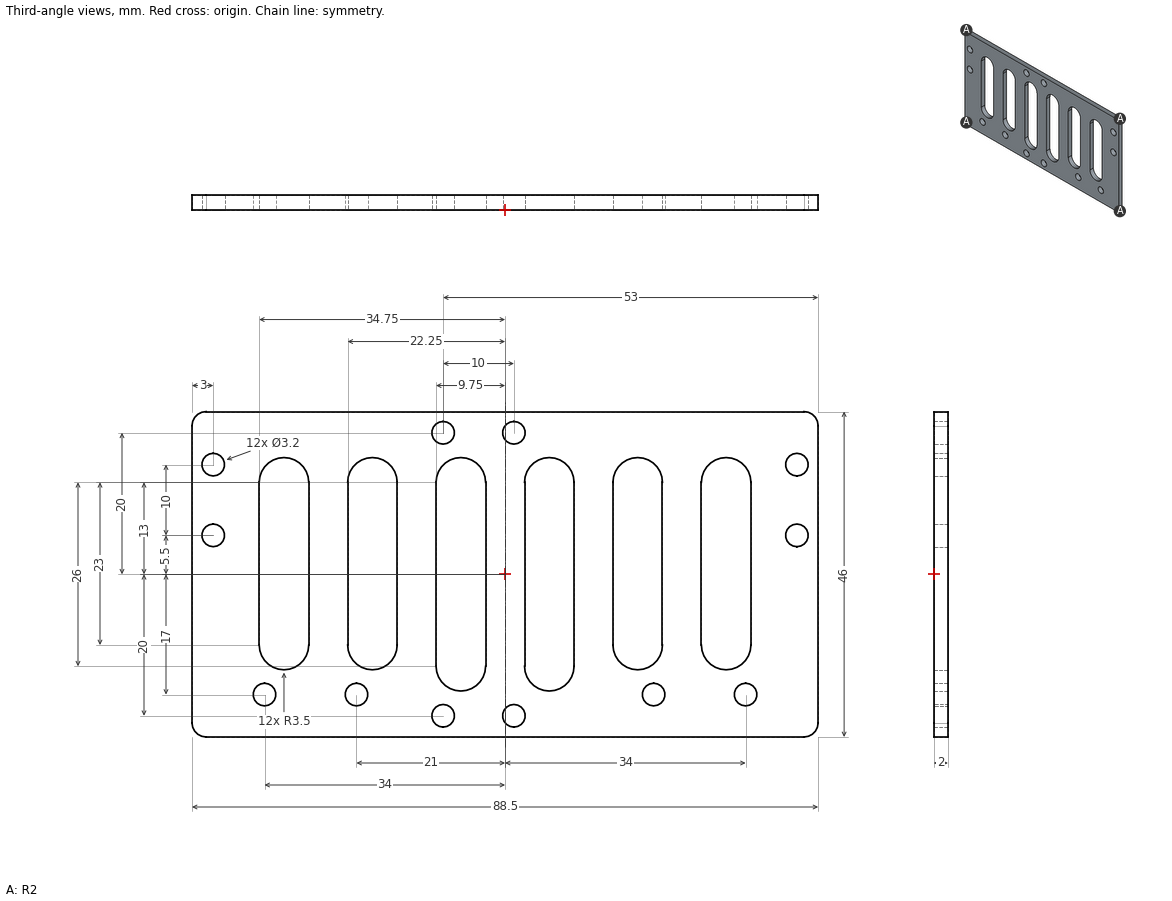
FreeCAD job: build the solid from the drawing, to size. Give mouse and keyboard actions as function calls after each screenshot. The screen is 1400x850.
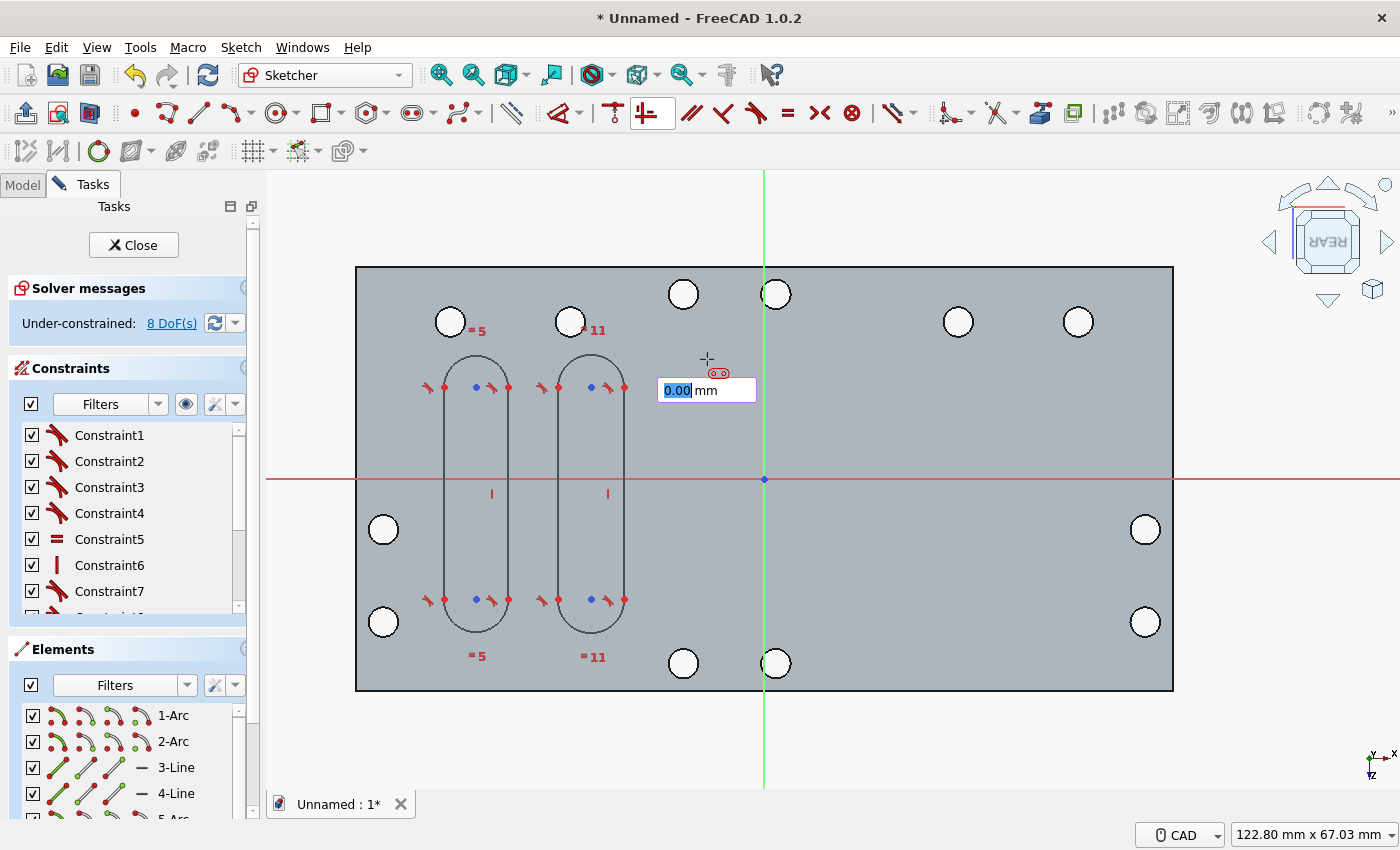
click(739, 515)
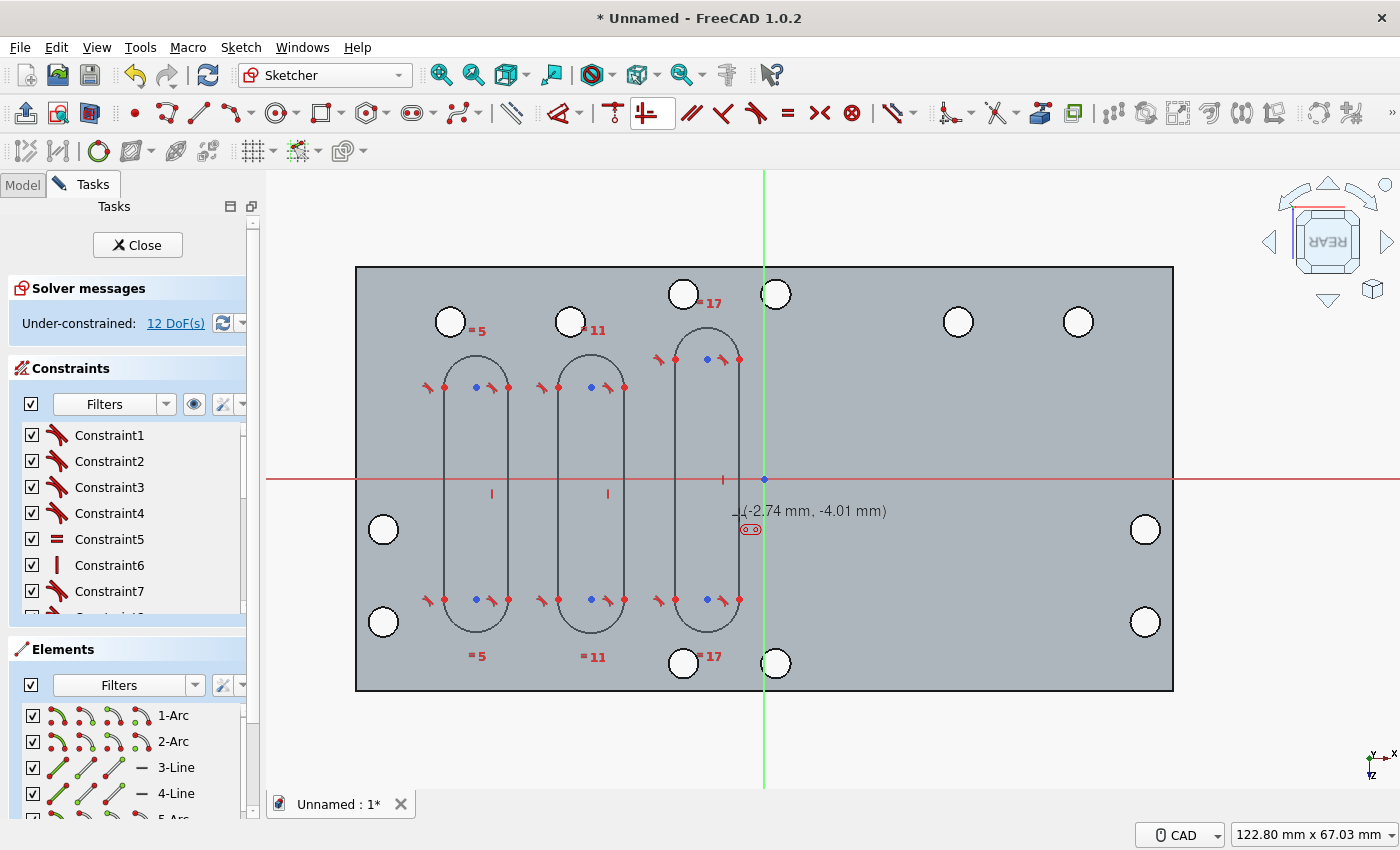
click(822, 599)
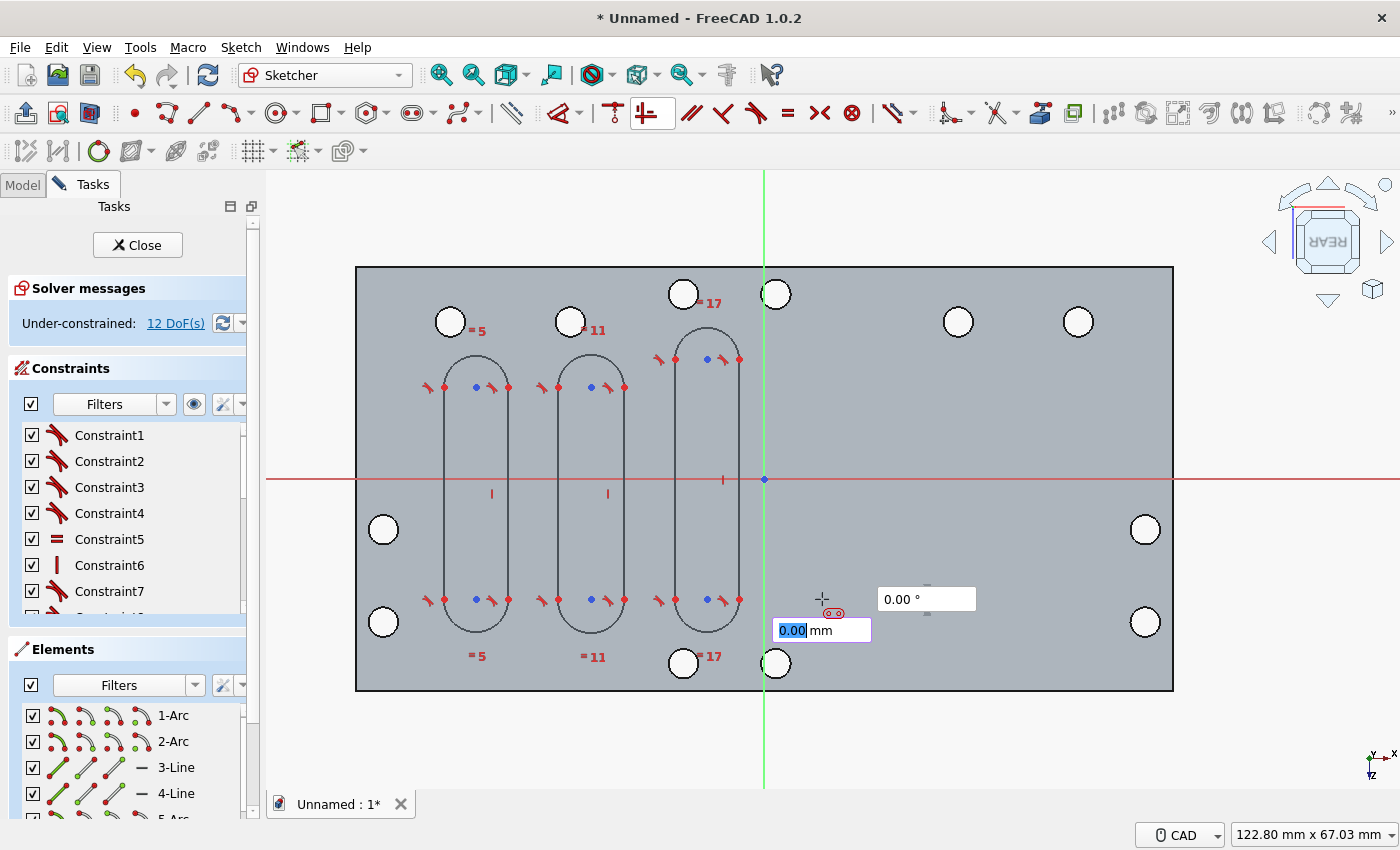
click(822, 359)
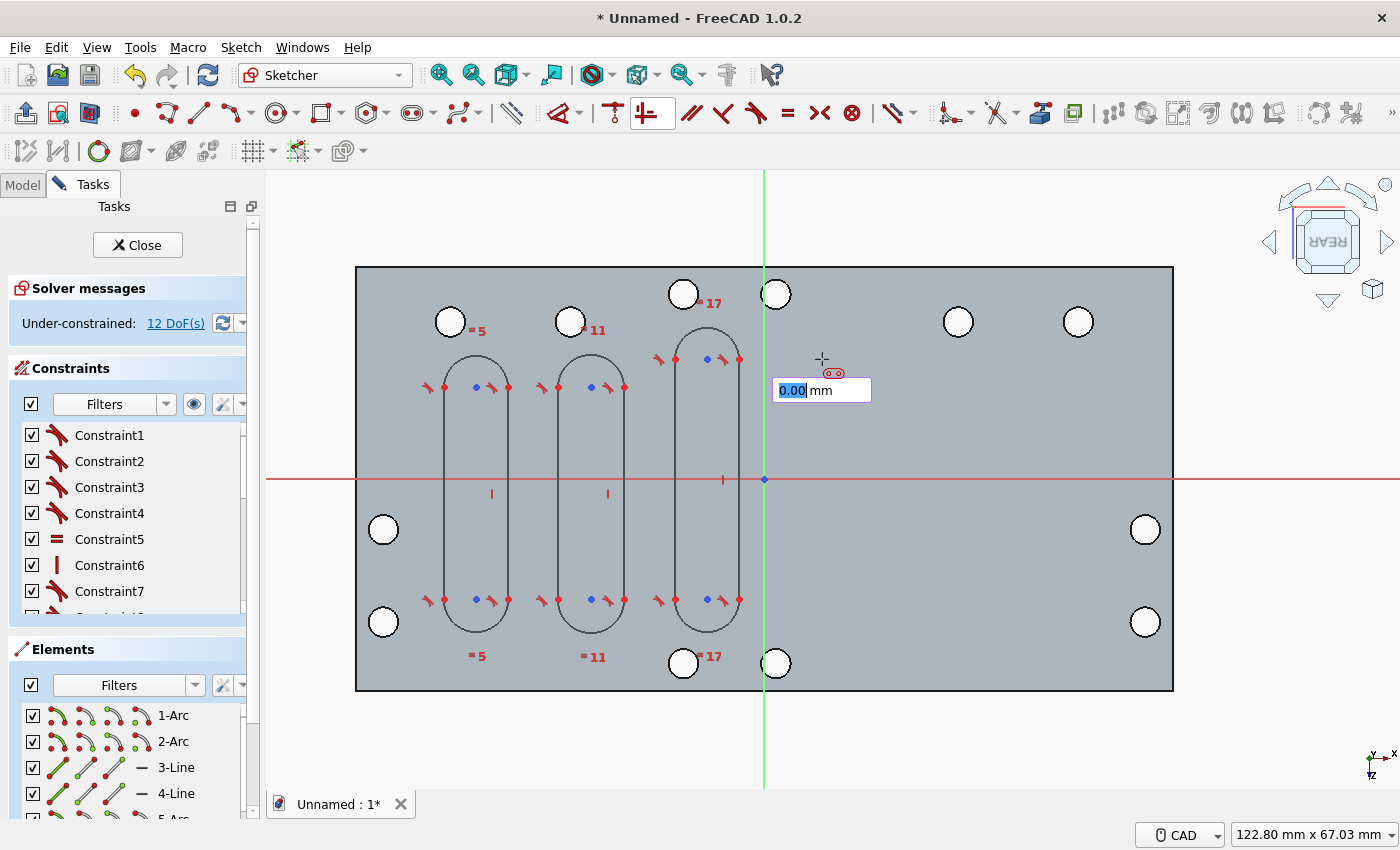
click(854, 515)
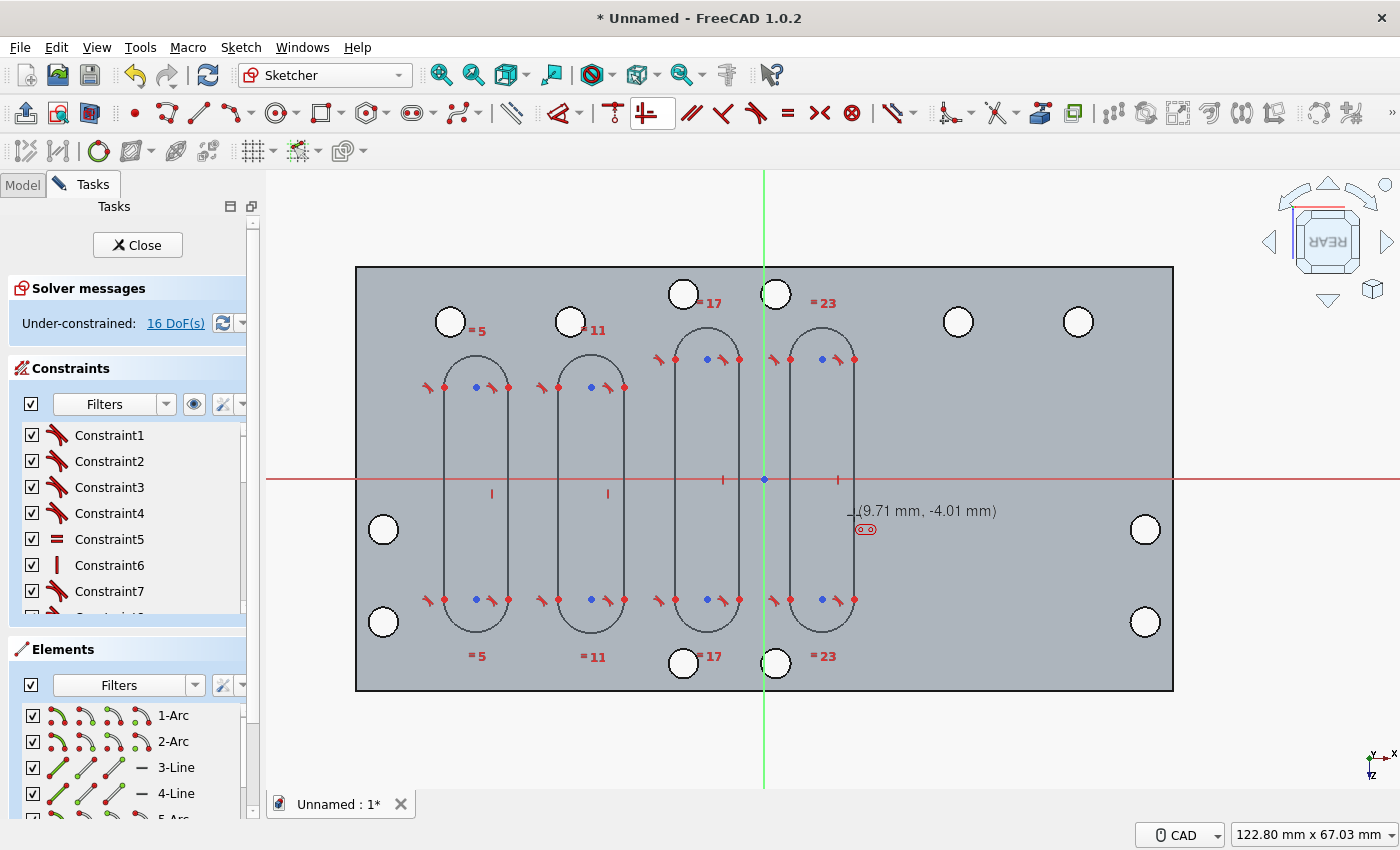
click(937, 599)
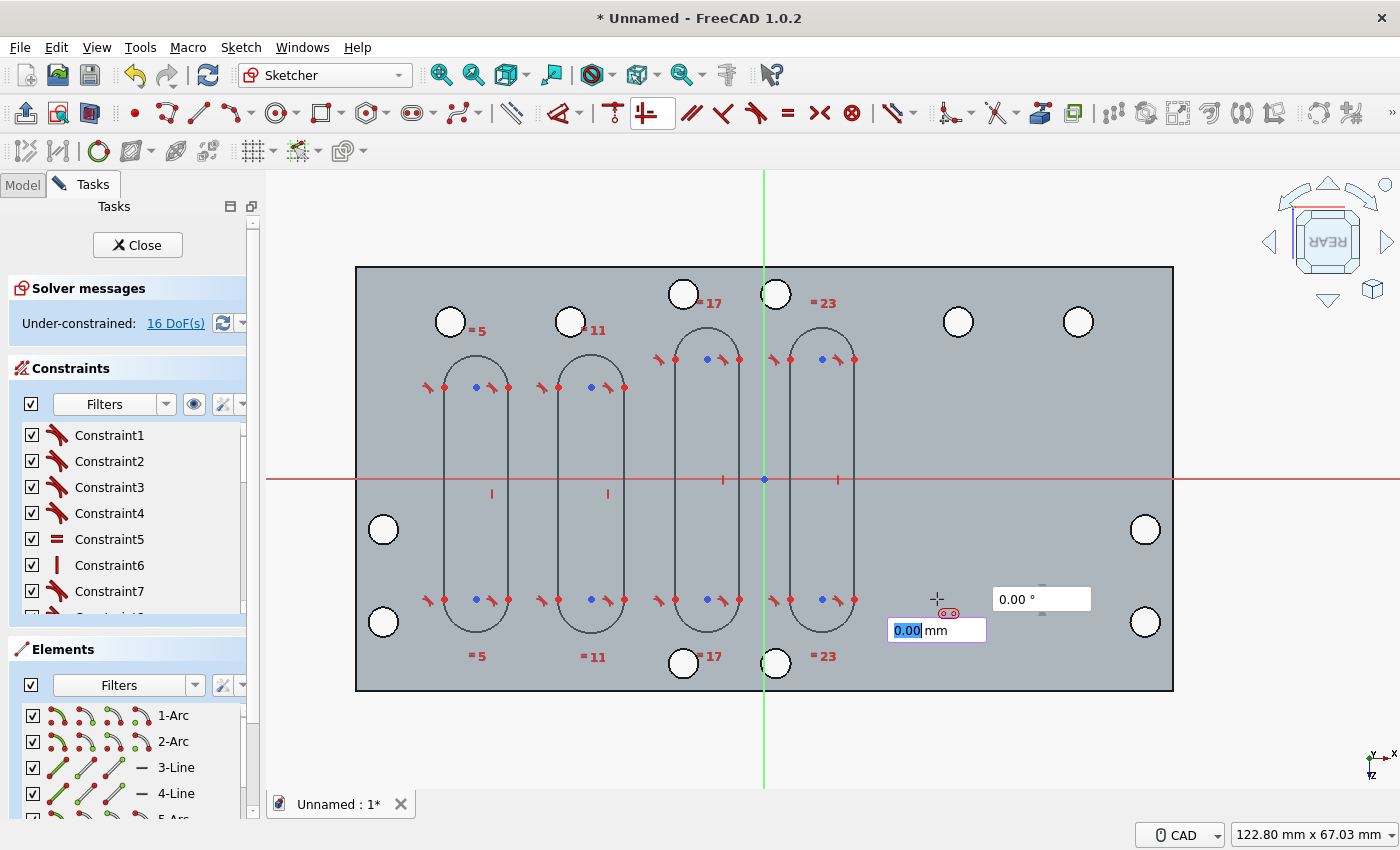
click(937, 387)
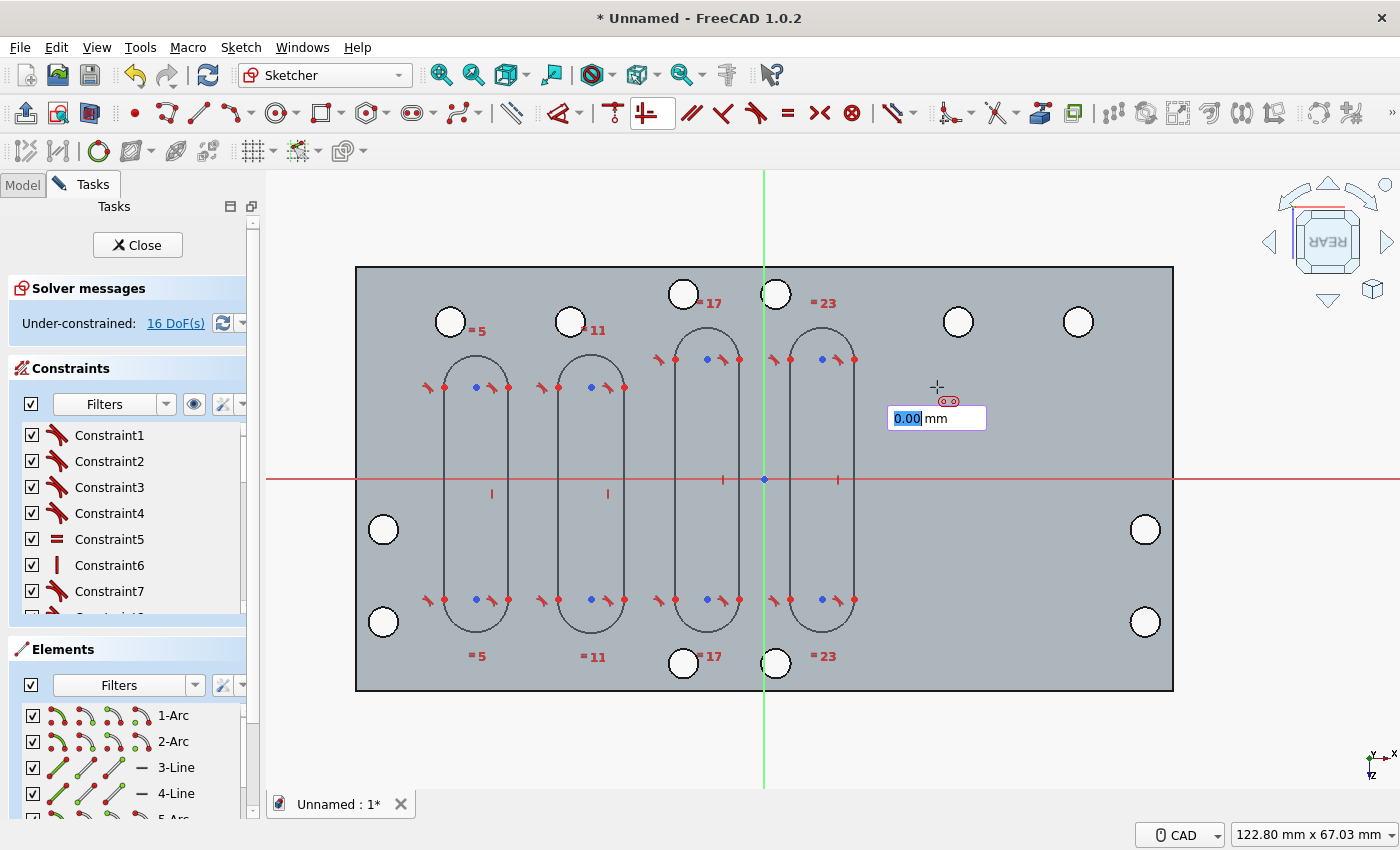
click(970, 525)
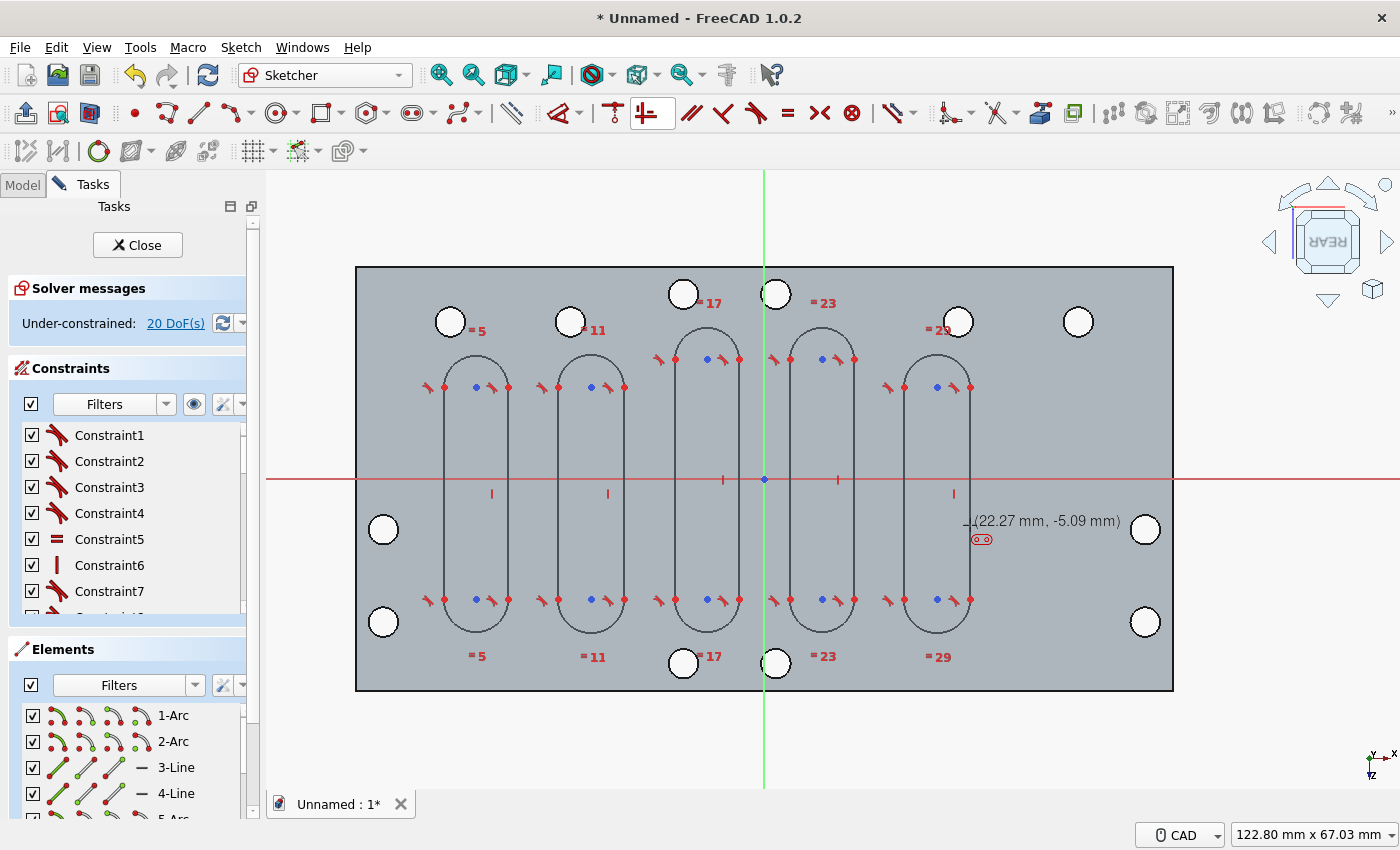
click(1053, 599)